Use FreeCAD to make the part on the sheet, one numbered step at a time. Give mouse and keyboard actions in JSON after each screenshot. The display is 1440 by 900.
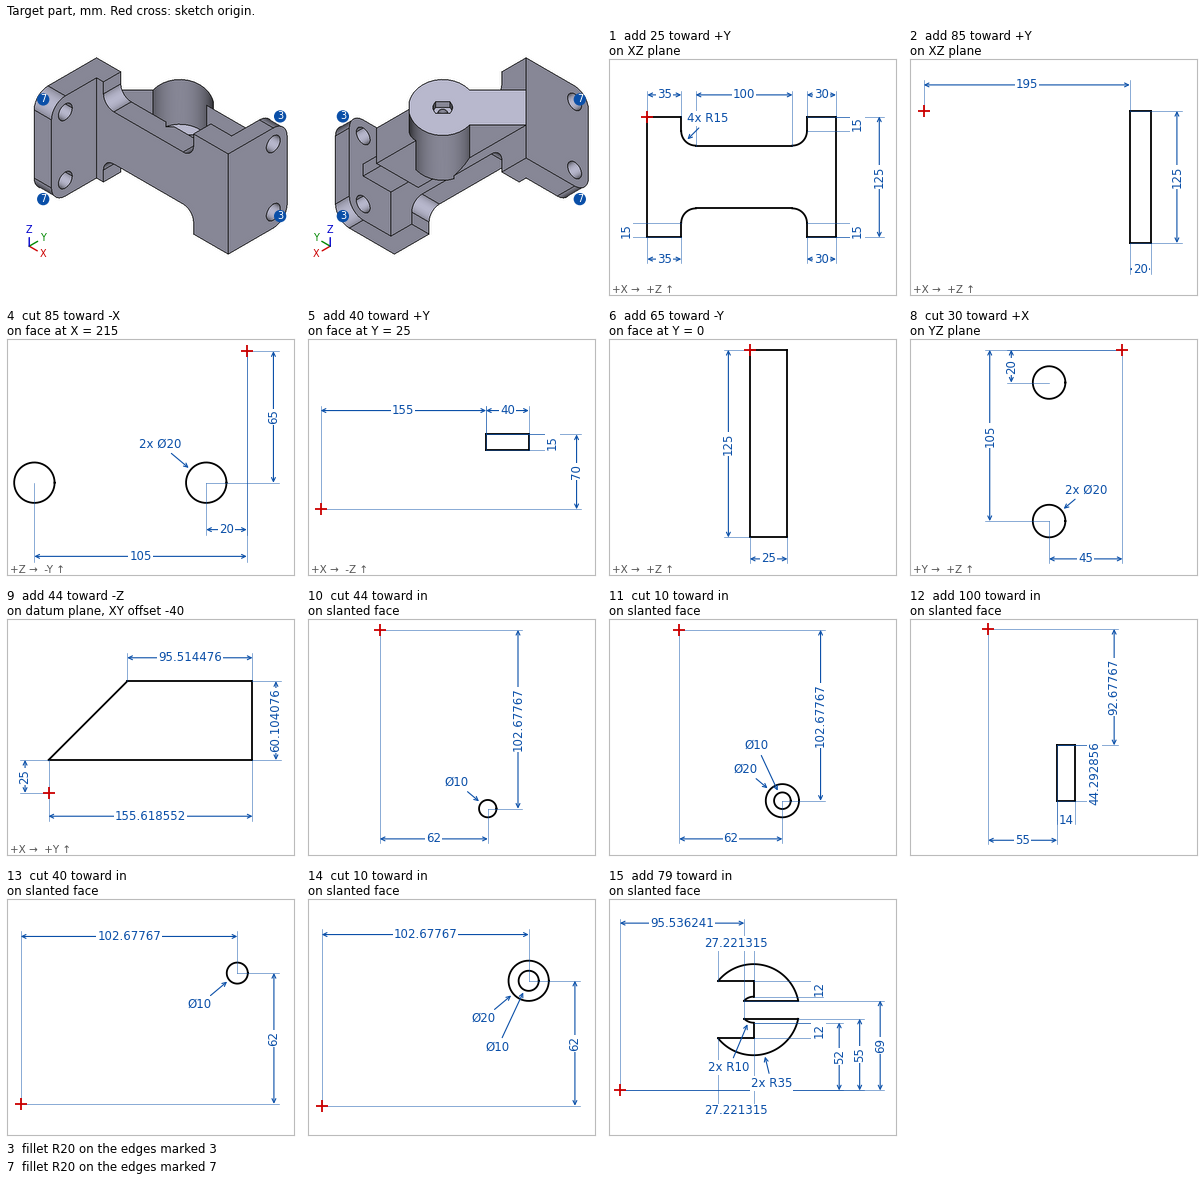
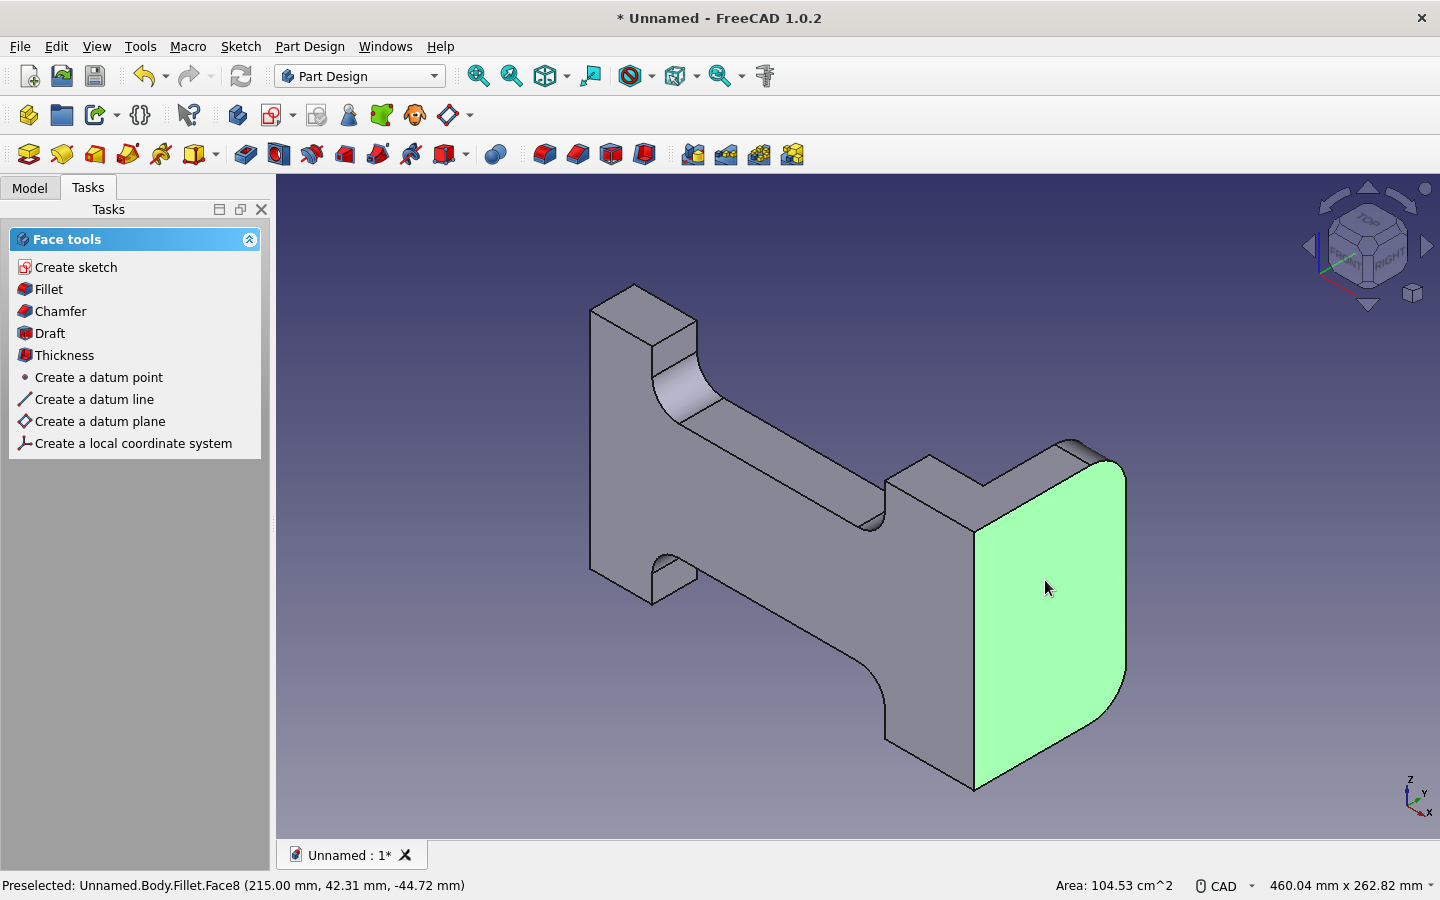
{"action": "left_click", "coordinate": [270, 116]}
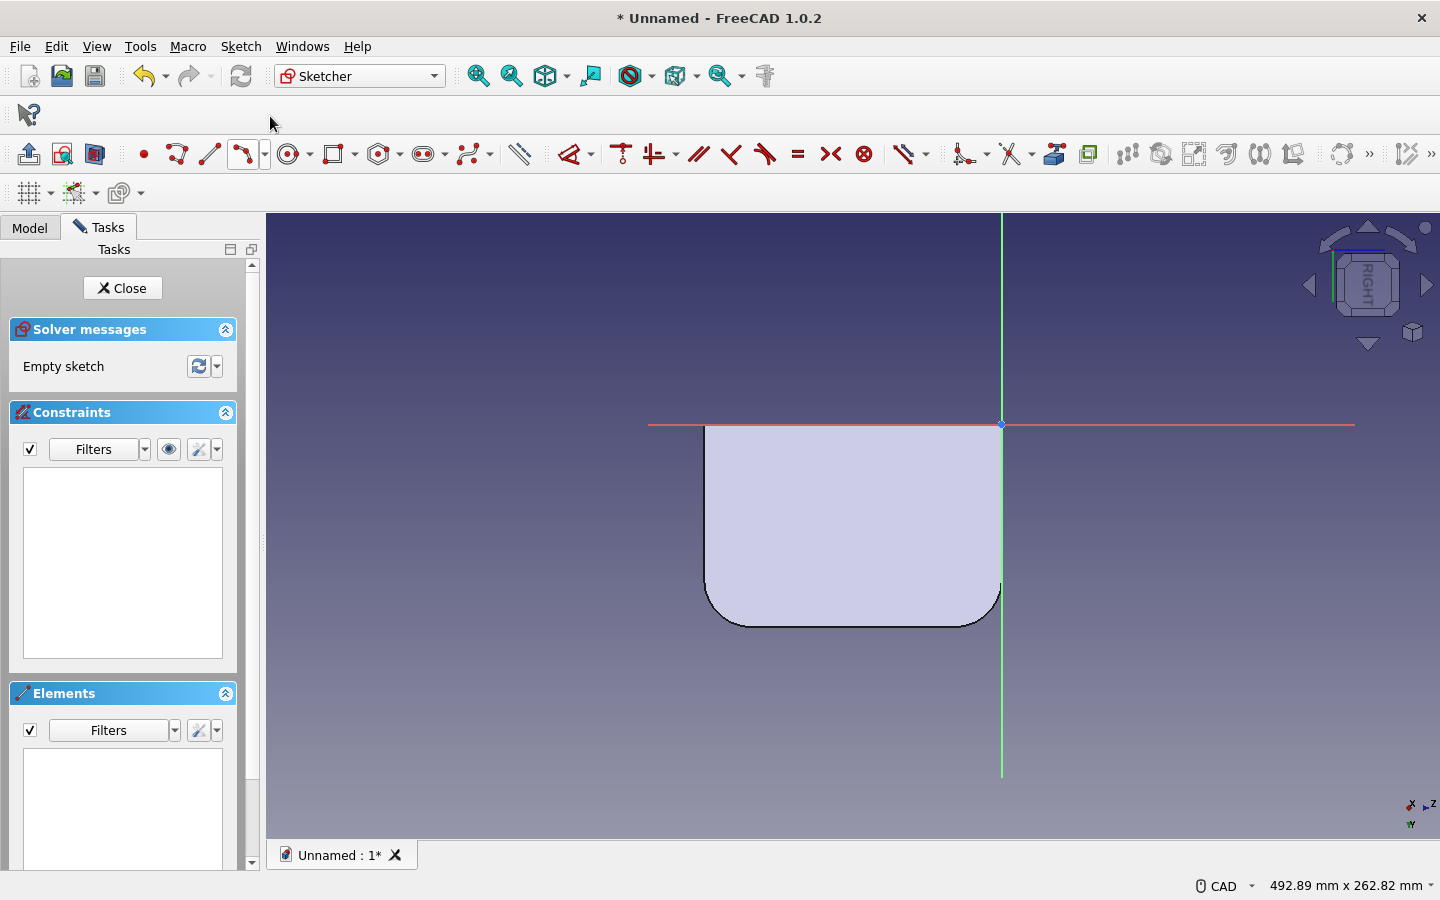
{"action": "scroll", "coordinate": [931, 504], "scroll_direction": "up", "scroll_amount": 4}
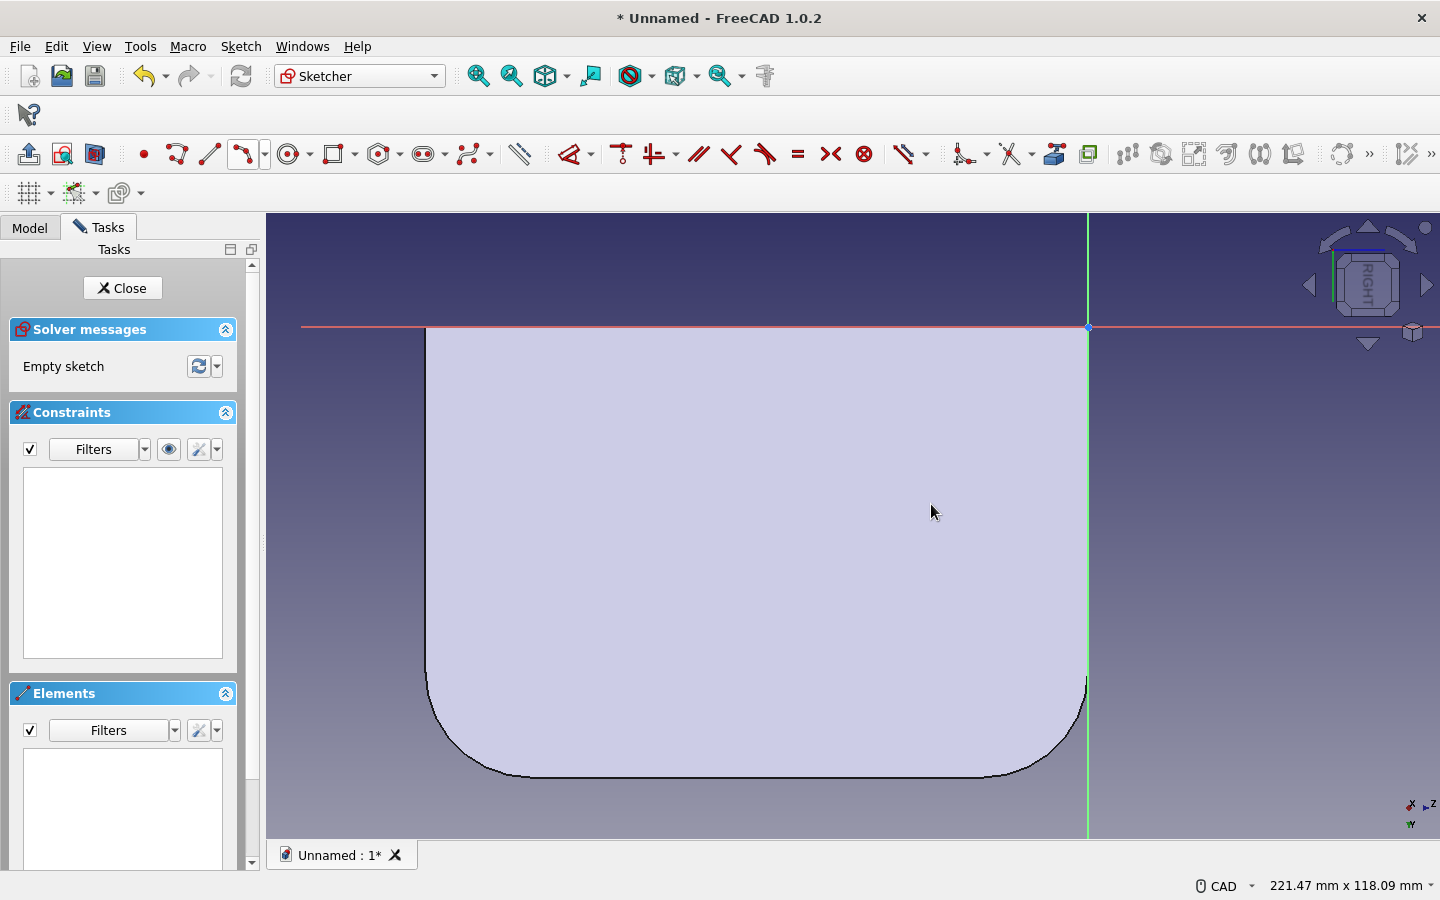
{"action": "left_click", "coordinate": [288, 154]}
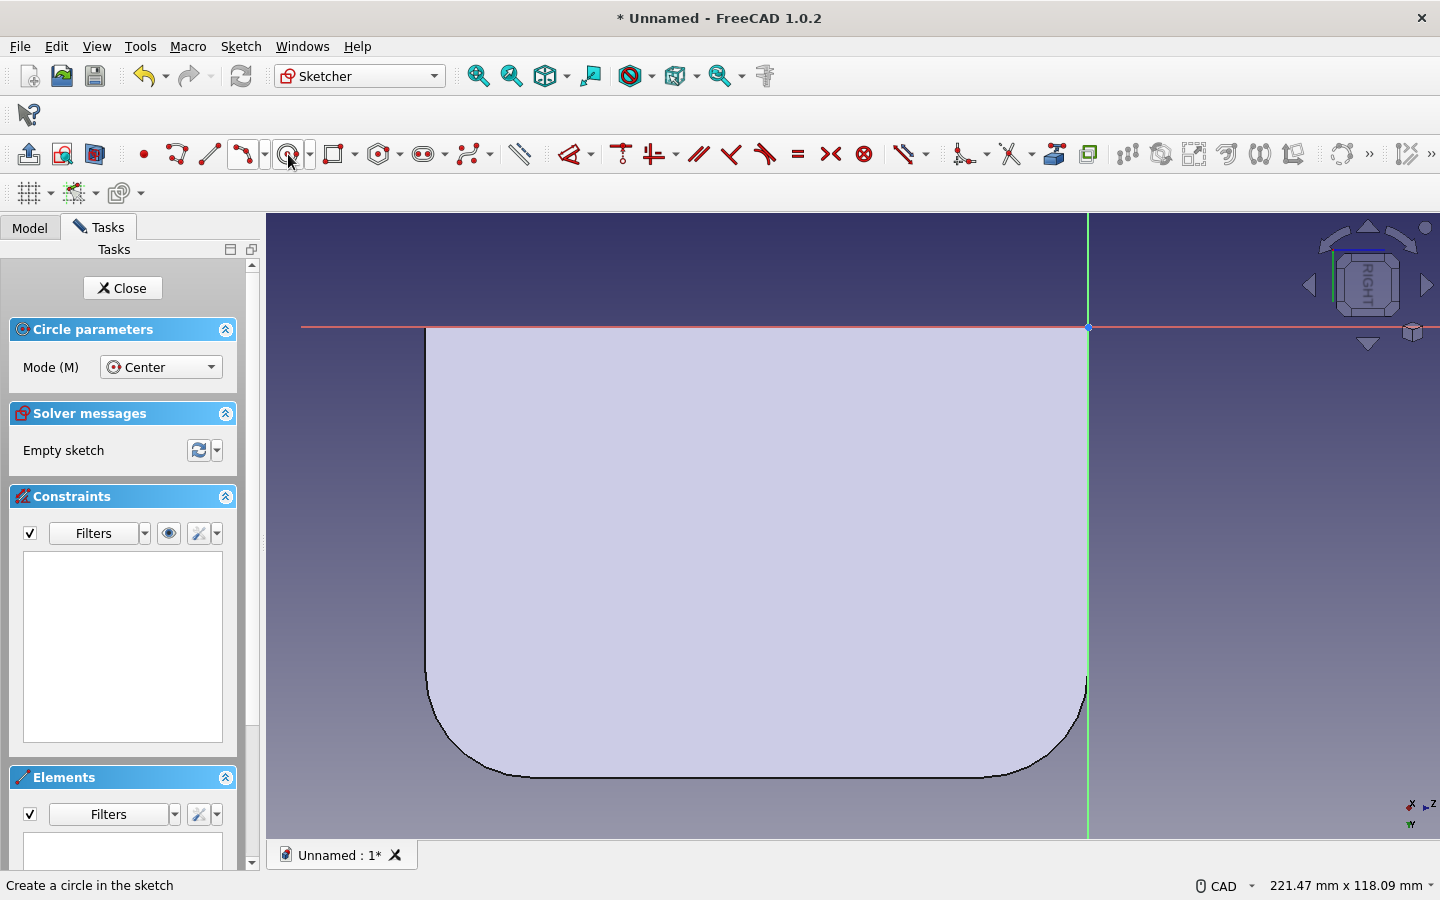
{"action": "left_click", "coordinate": [982, 672]}
{"action": "left_click", "coordinate": [1019, 634]}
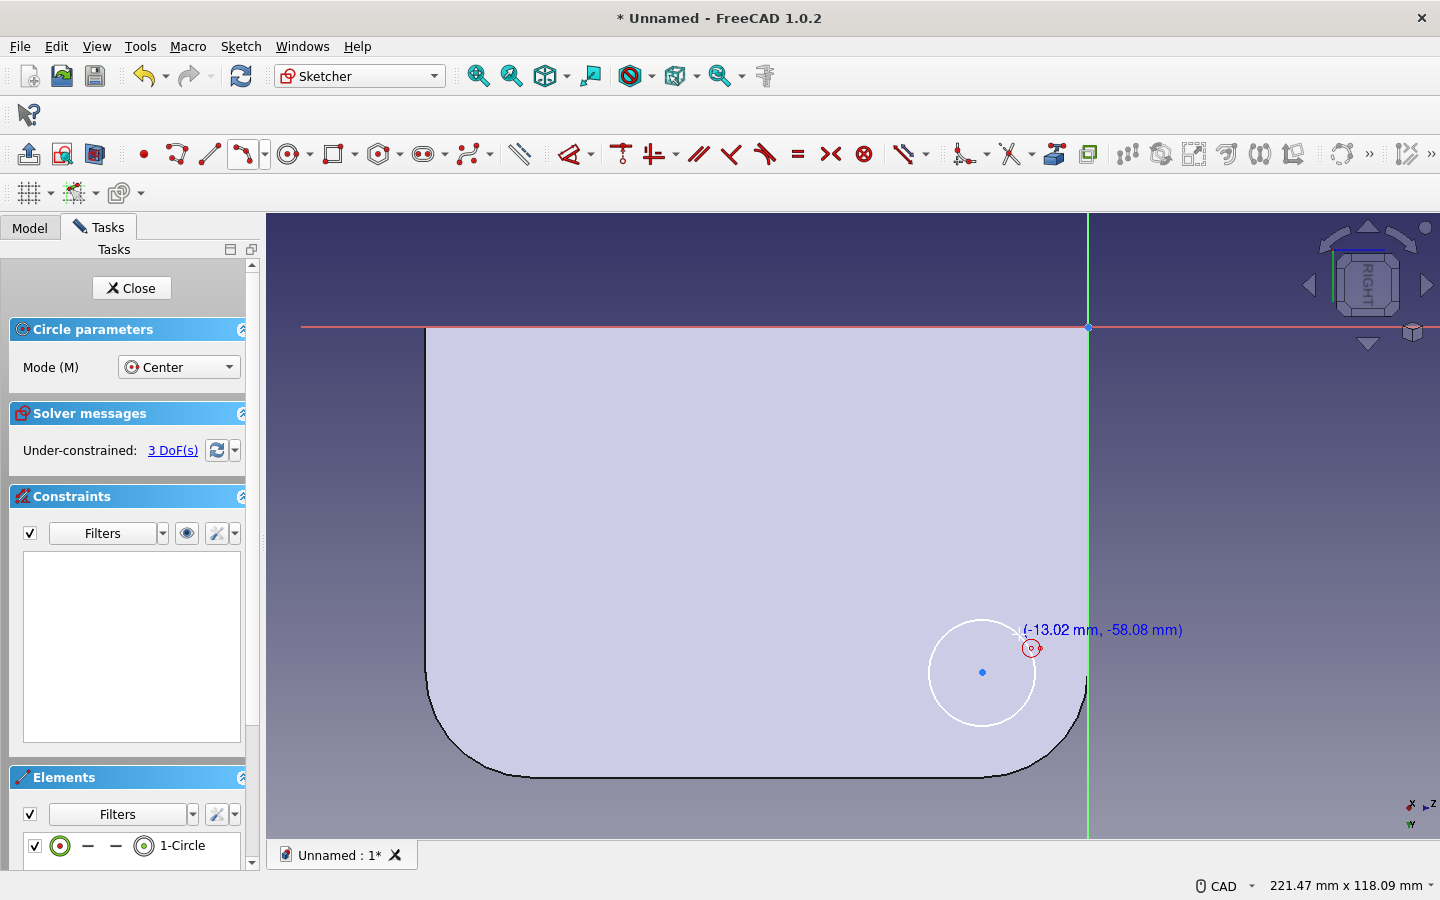
{"action": "left_click", "coordinate": [531, 672]}
{"action": "left_click", "coordinate": [569, 634]}
{"action": "key", "text": "Escape"}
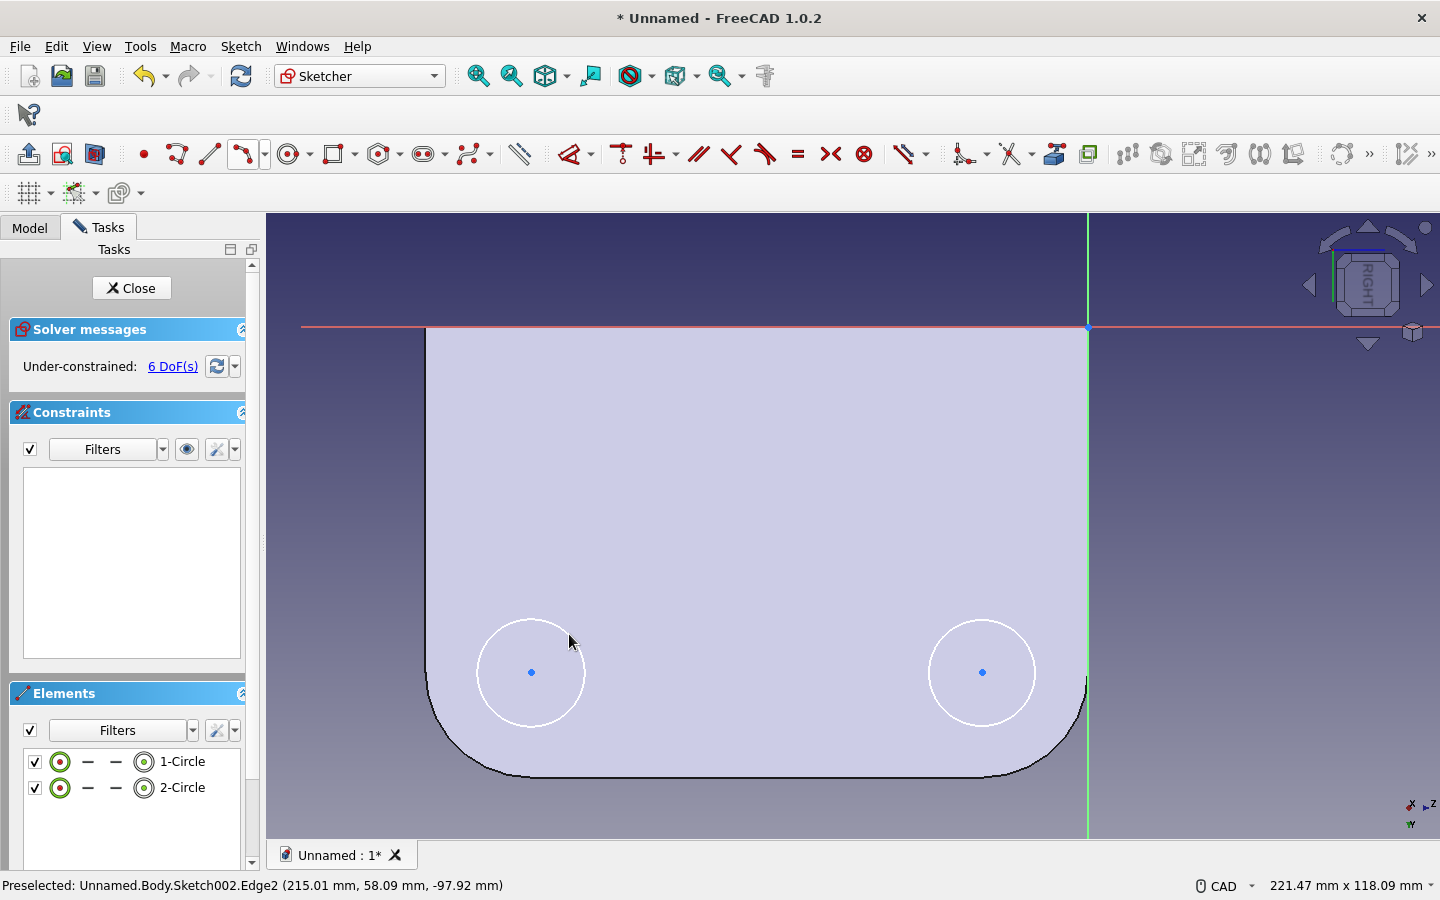
{"action": "left_click", "coordinate": [1019, 635]}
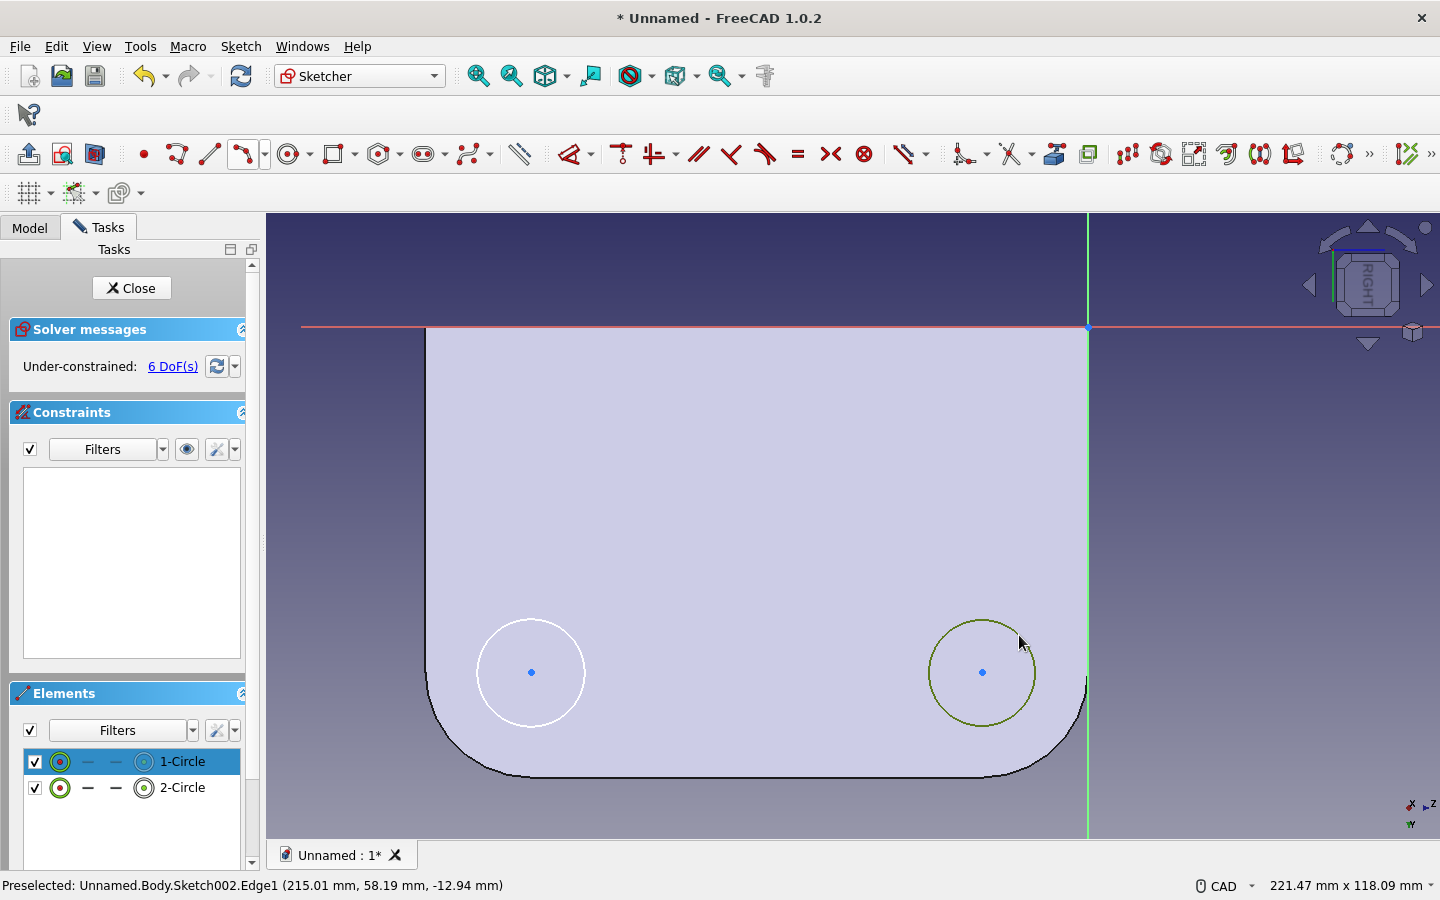
{"action": "left_click", "coordinate": [569, 635]}